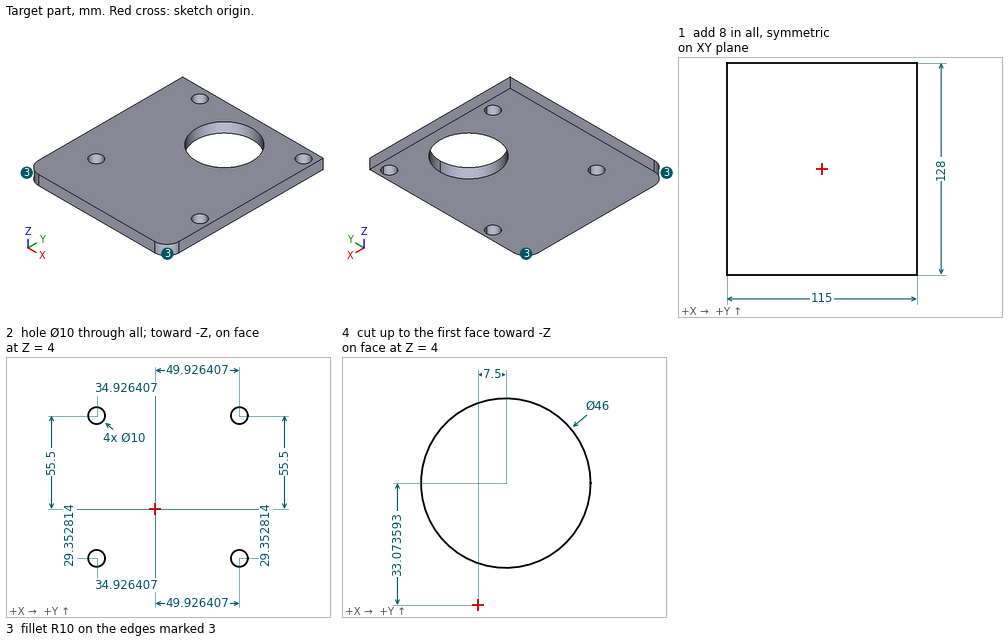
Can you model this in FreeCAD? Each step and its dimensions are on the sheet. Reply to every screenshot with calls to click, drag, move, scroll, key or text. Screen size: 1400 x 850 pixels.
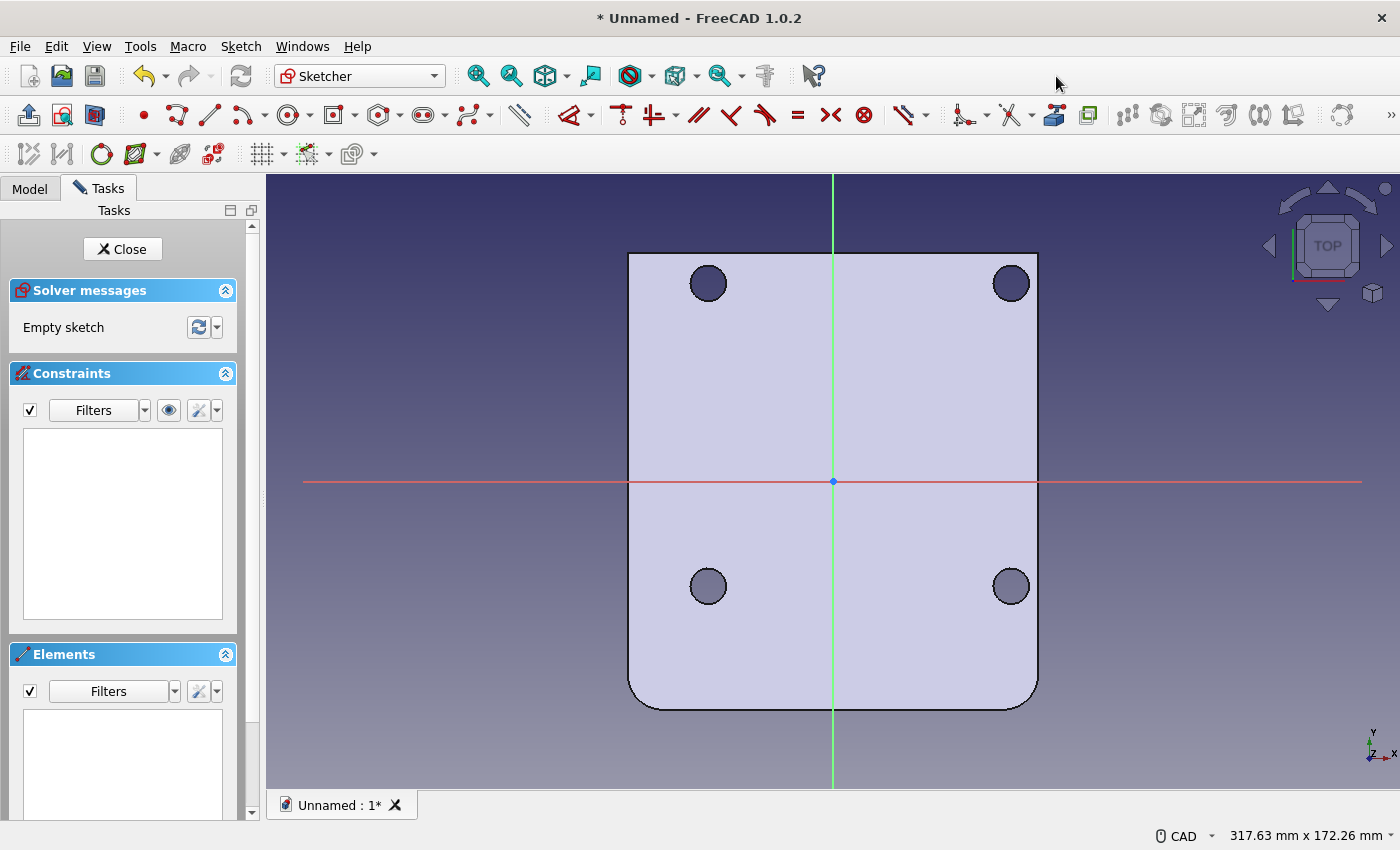
scroll(976, 260, up, 3)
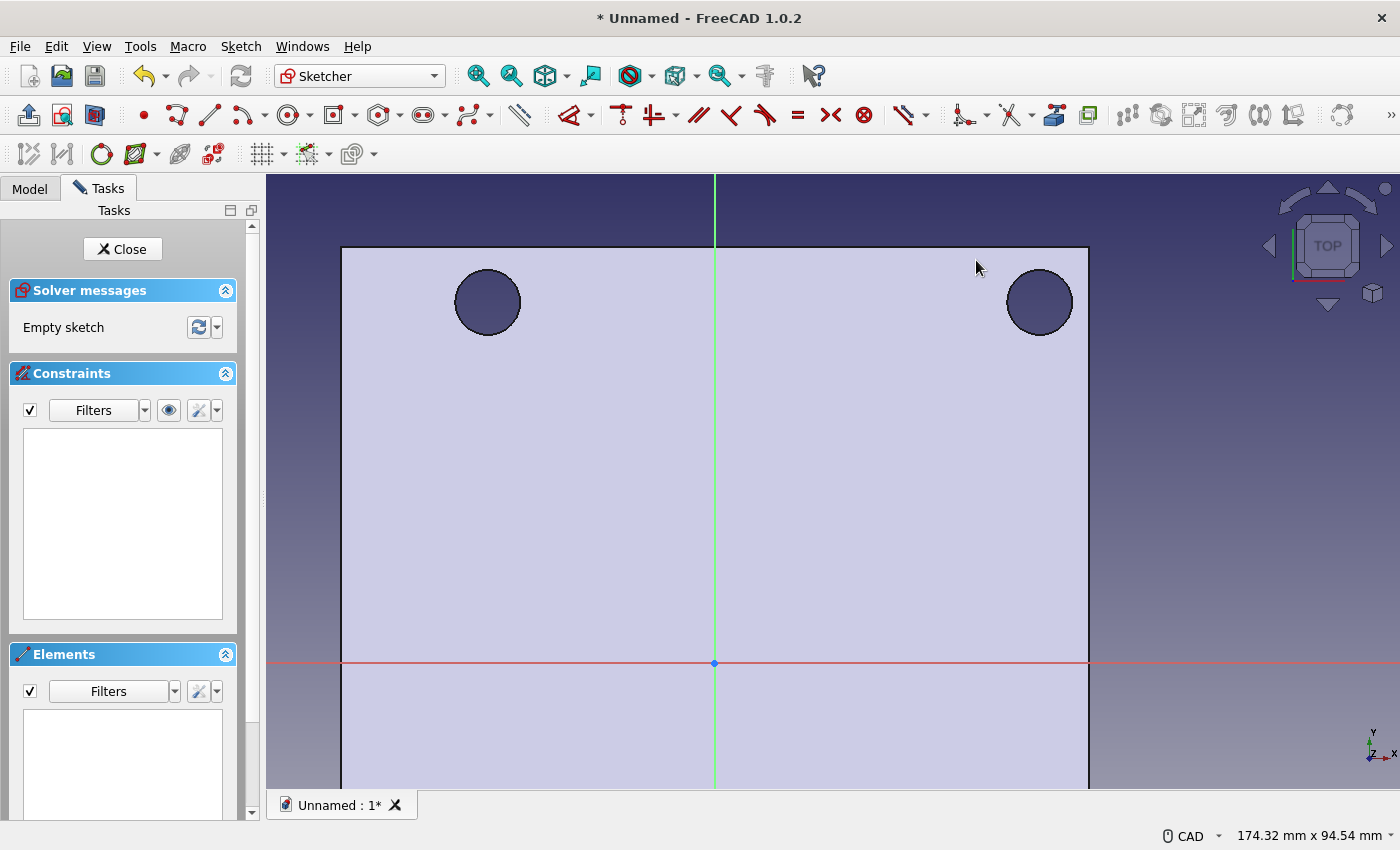
click(288, 116)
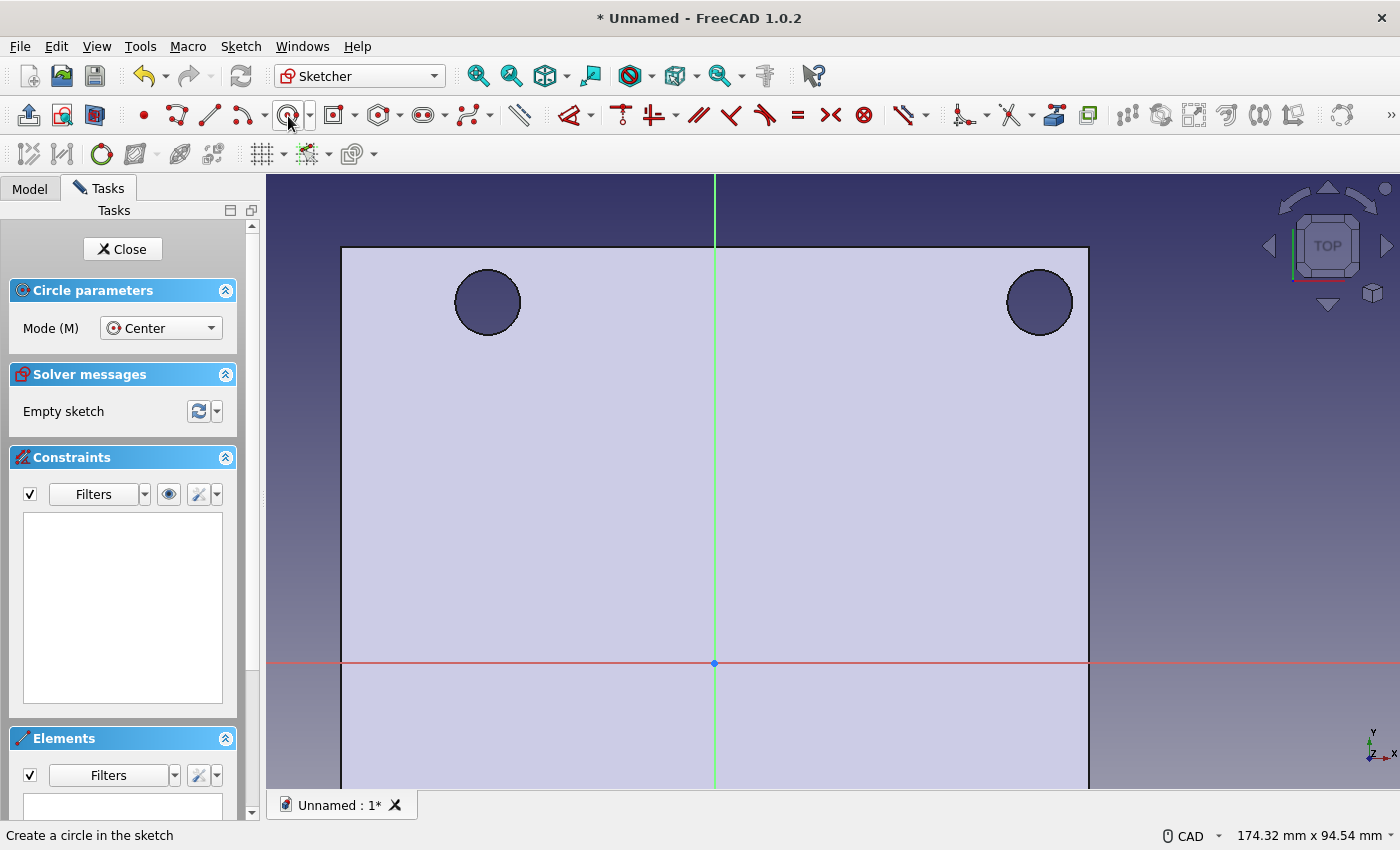
click(764, 448)
move(870, 343)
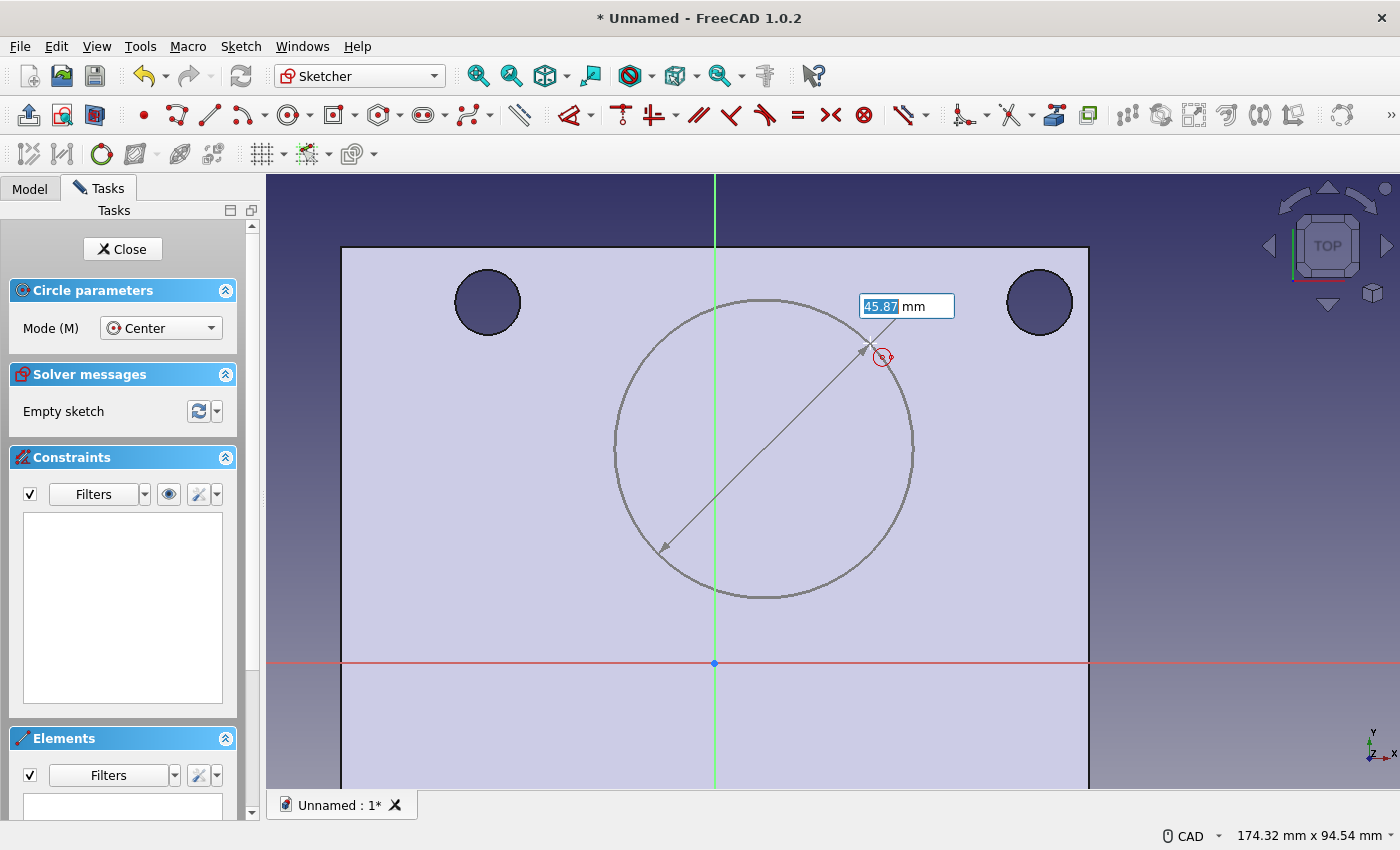
text(46)
key(Return)
key(Escape)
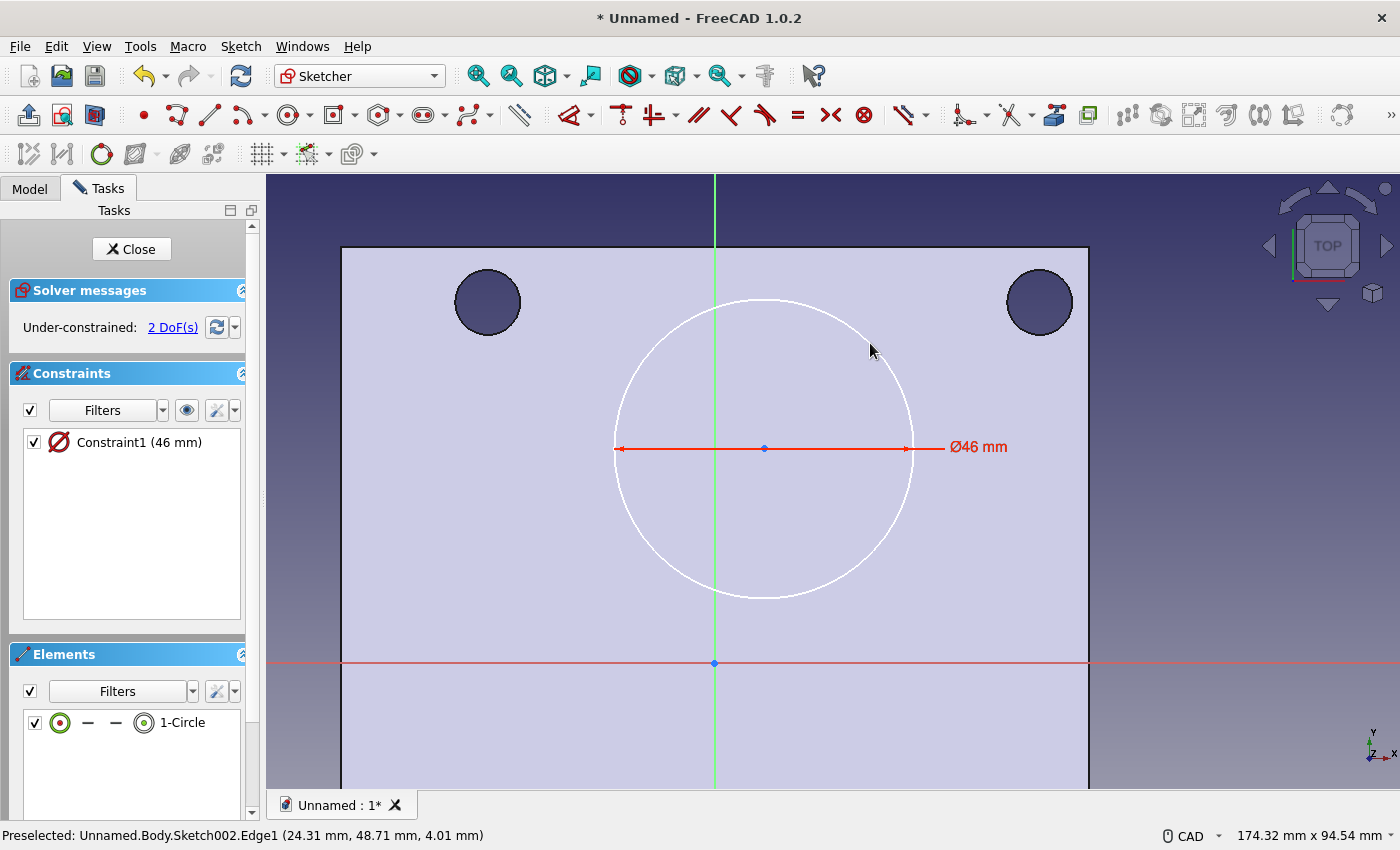
click(568, 116)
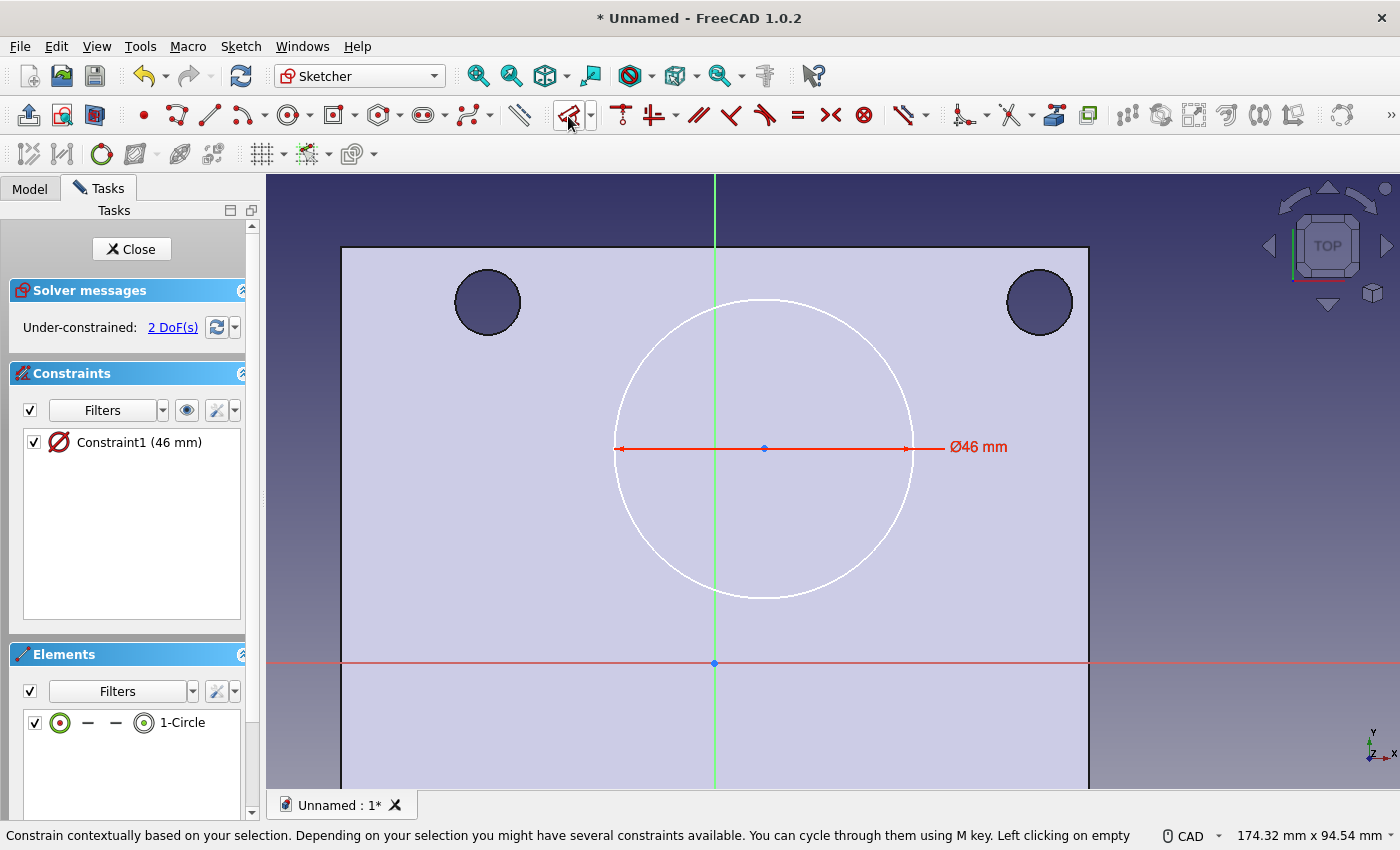
click(764, 449)
click(739, 697)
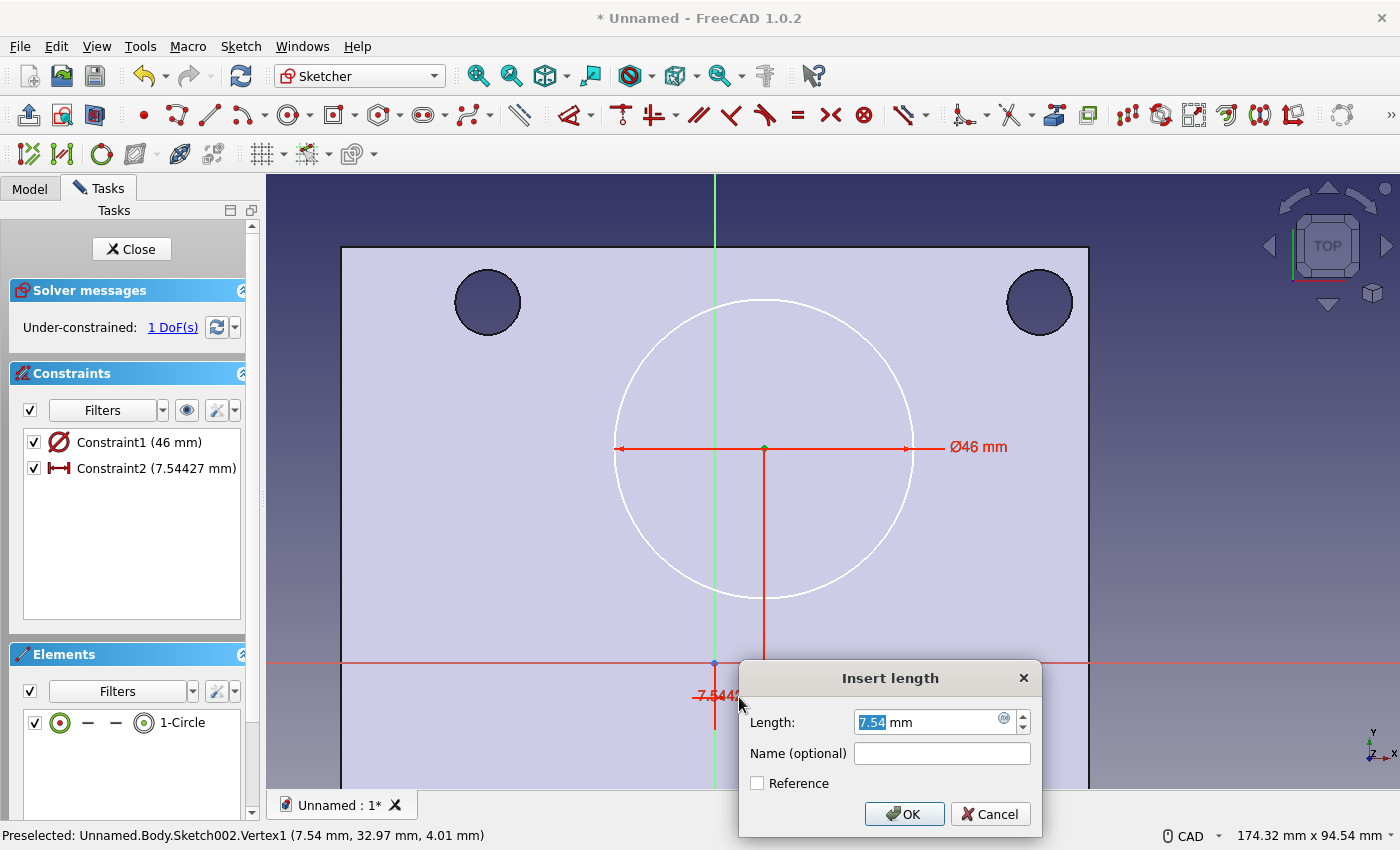
text(7.5)
key(Return)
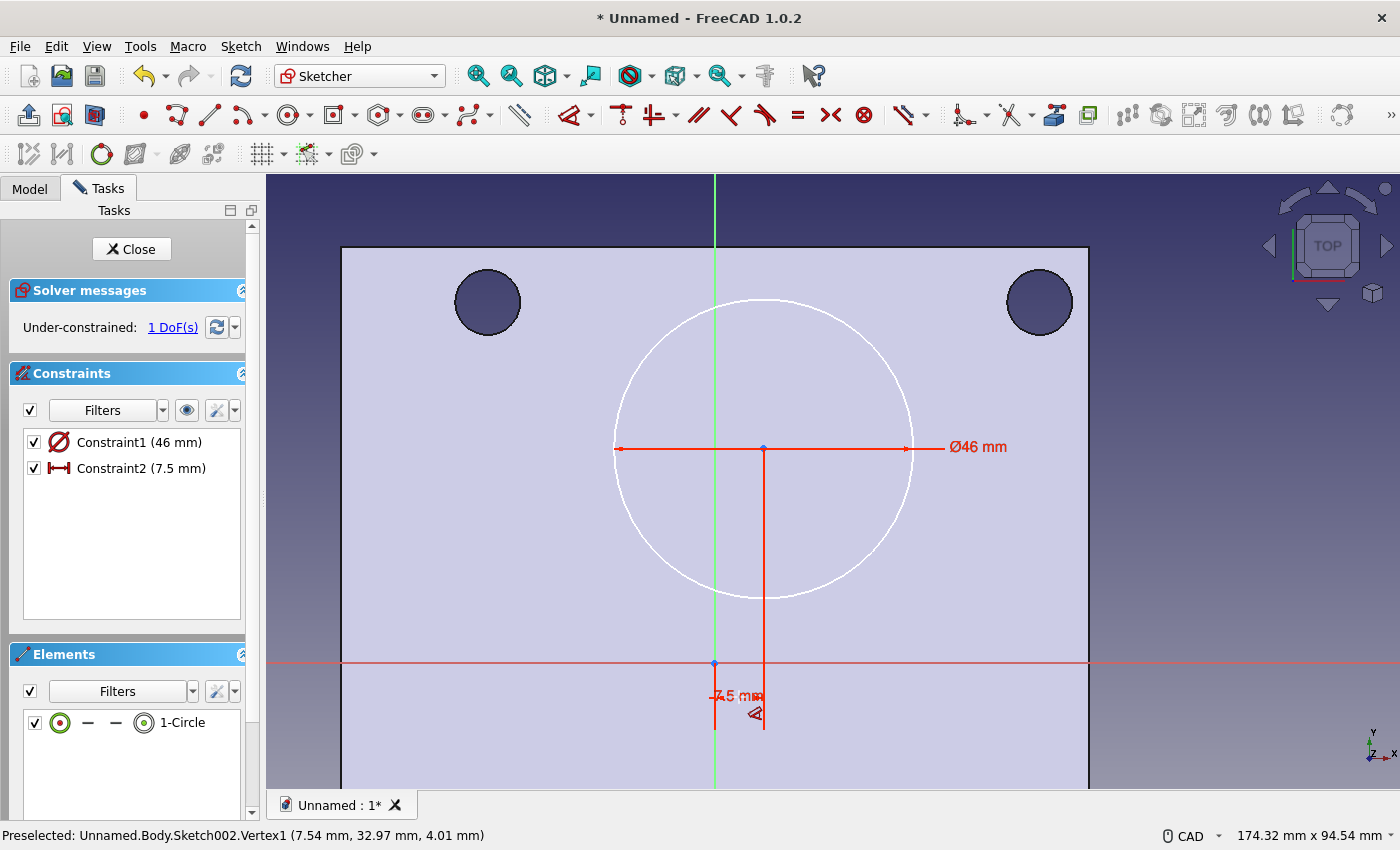
click(764, 449)
click(681, 556)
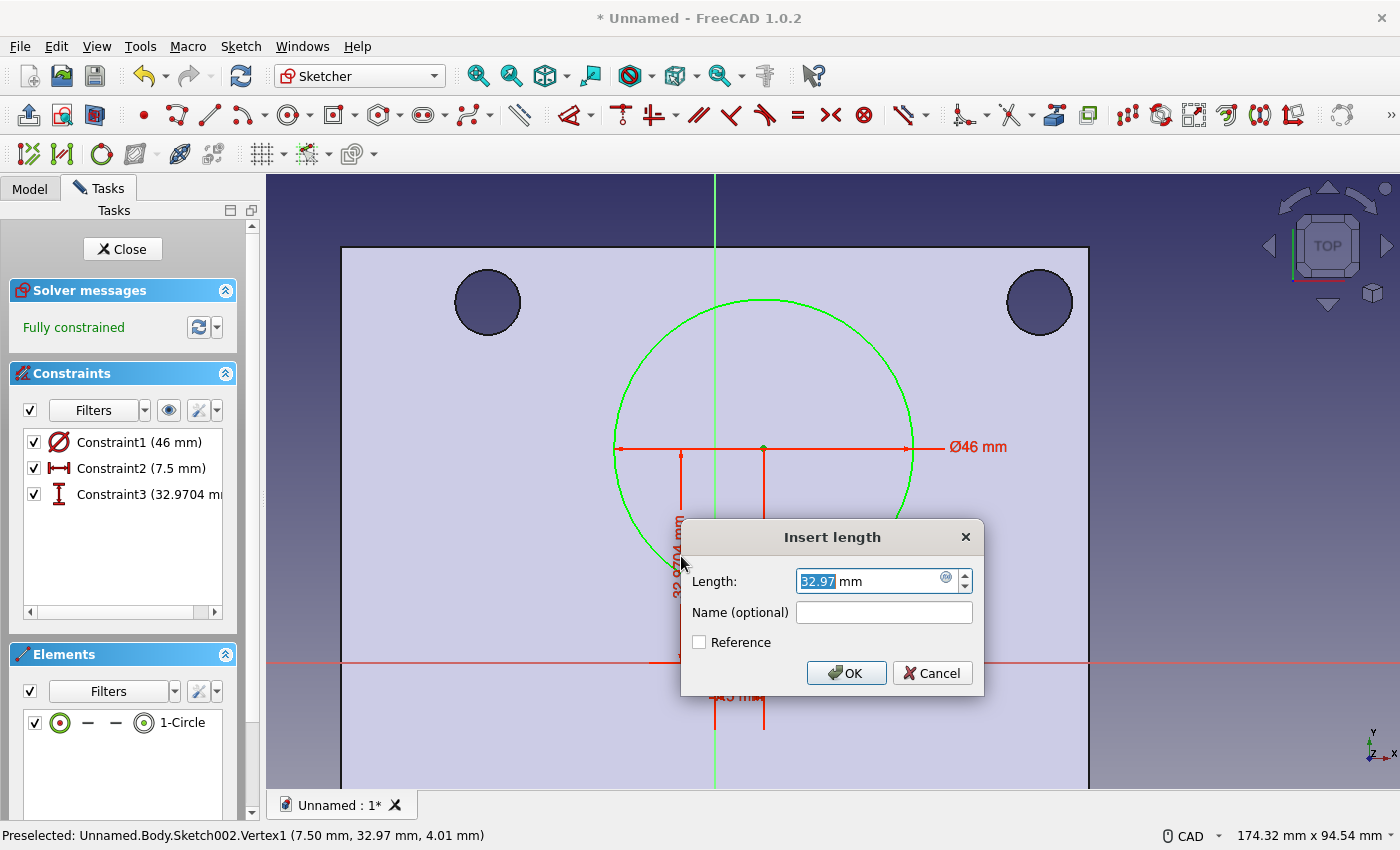
text(33.073593)
key(Return)
key(Escape)